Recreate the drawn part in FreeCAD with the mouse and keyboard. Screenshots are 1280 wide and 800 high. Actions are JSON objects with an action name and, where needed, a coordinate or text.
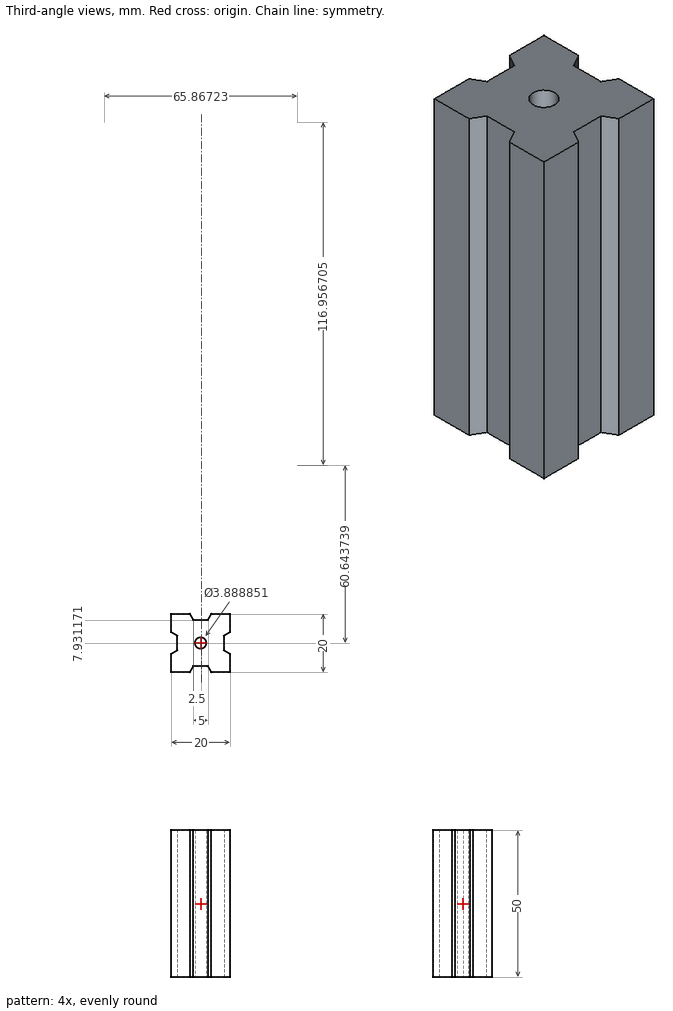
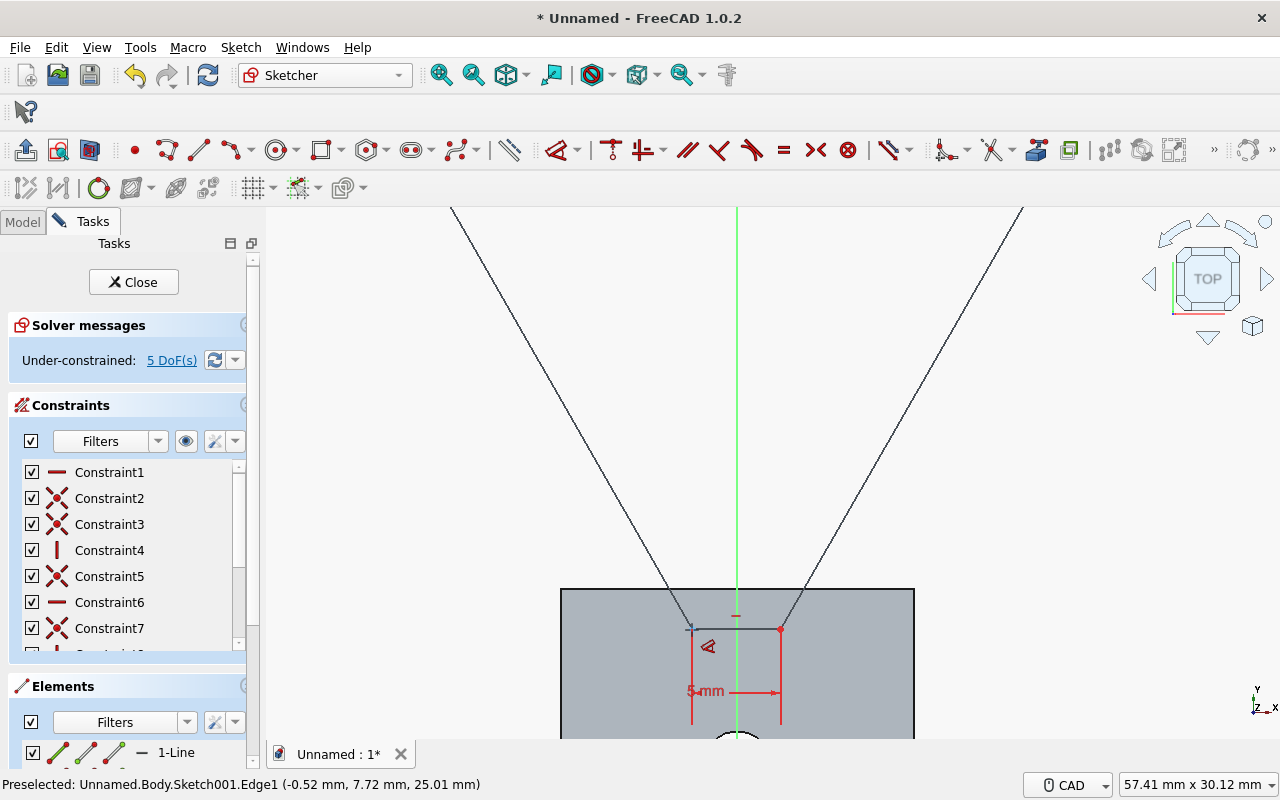
{"action": "left_click", "coordinate": [692, 629]}
{"action": "left_click", "coordinate": [715, 595]}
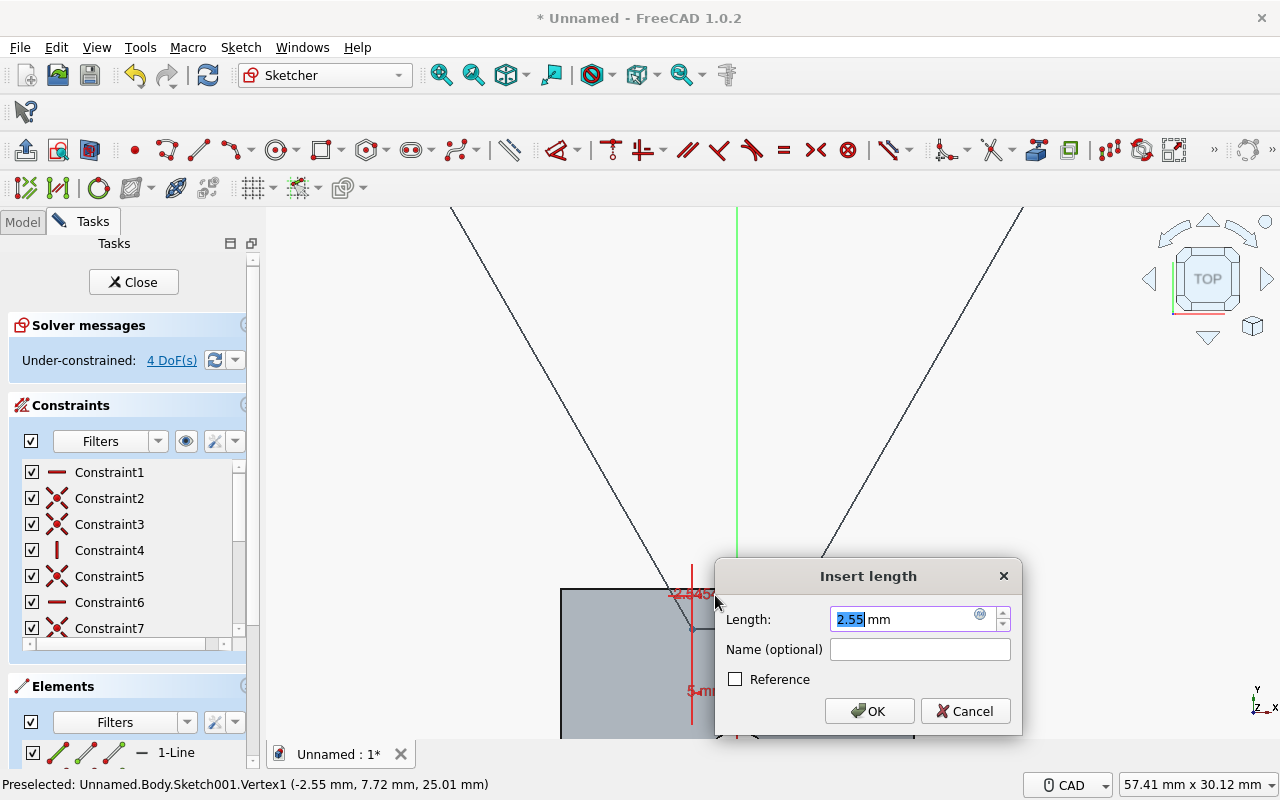
{"action": "type", "text": "2.5"}
{"action": "key", "text": "Return"}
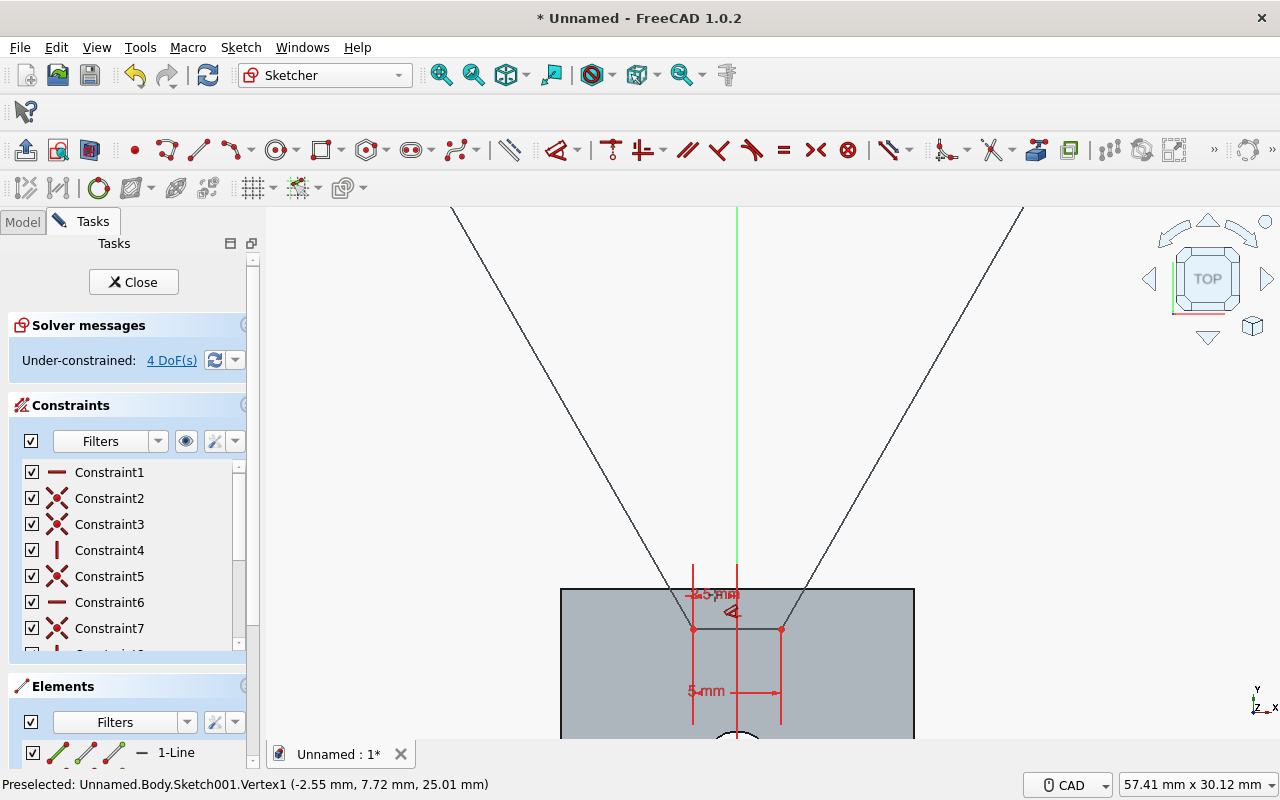
{"action": "scroll", "coordinate": [700, 632], "scroll_direction": "down", "scroll_amount": 11}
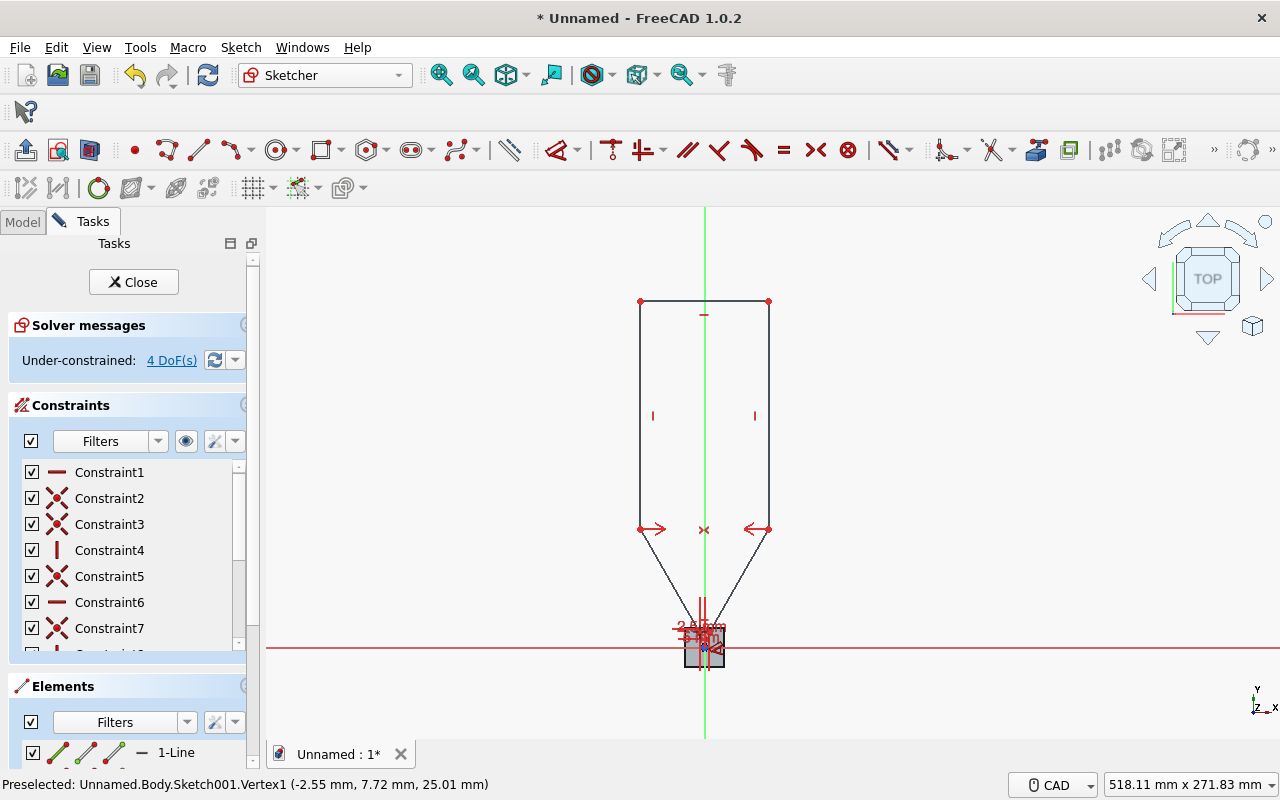
{"action": "left_click", "coordinate": [730, 301]}
{"action": "left_click", "coordinate": [675, 267]}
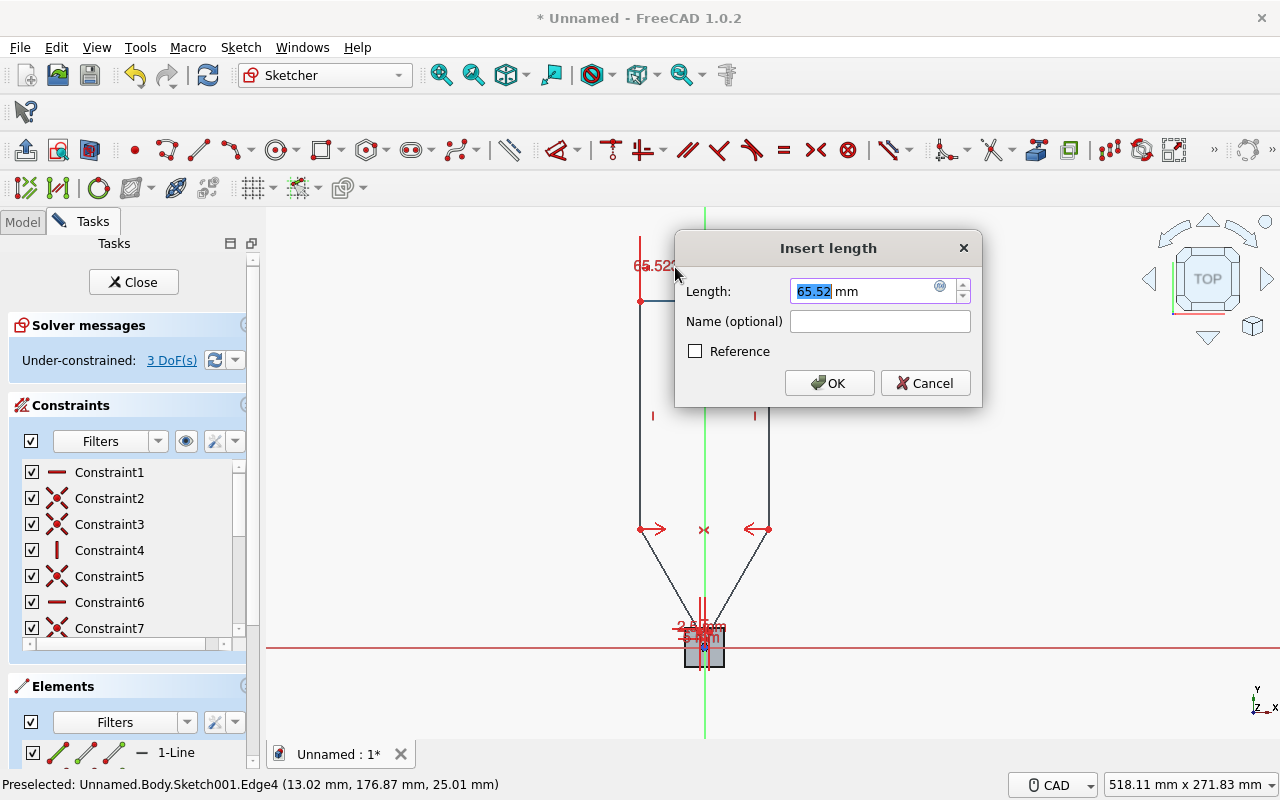
{"action": "type", "text": "65.86723"}
{"action": "key", "text": "Return"}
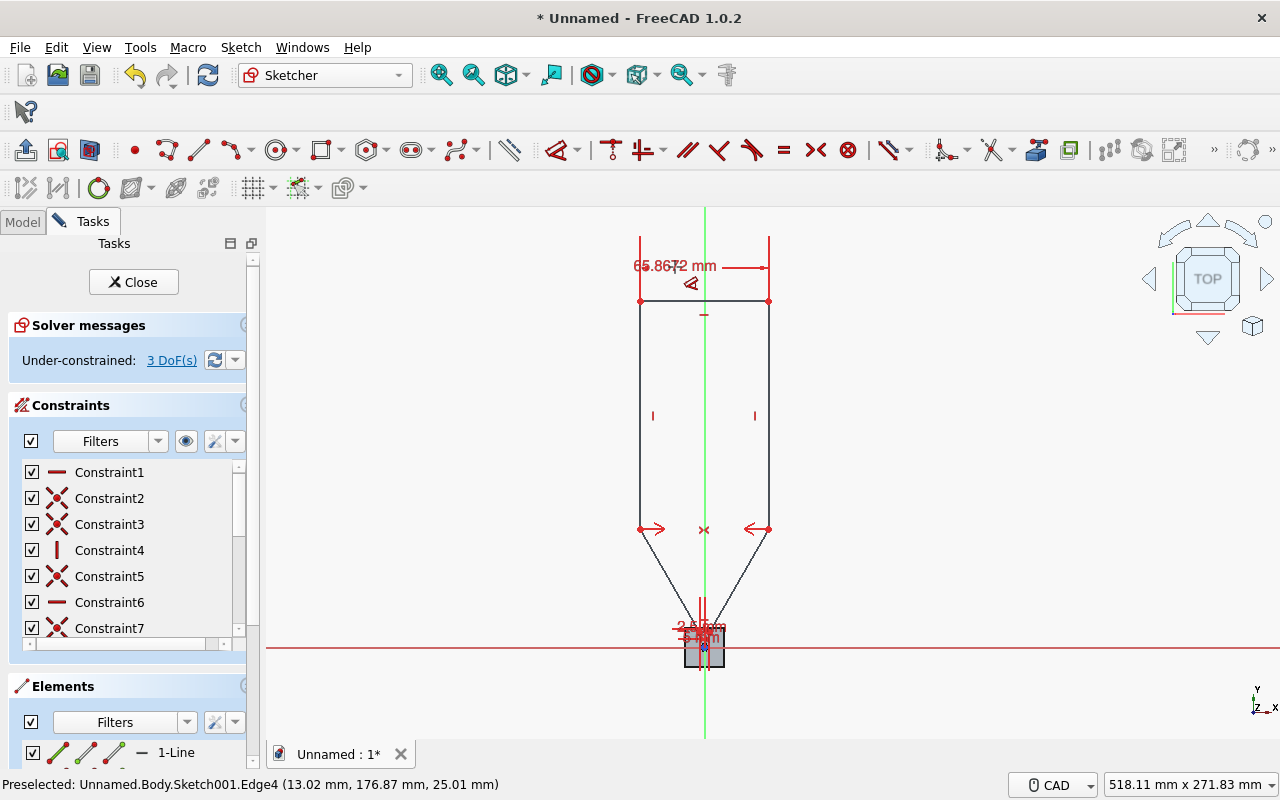
{"action": "scroll", "coordinate": [700, 632], "scroll_direction": "up", "scroll_amount": 5}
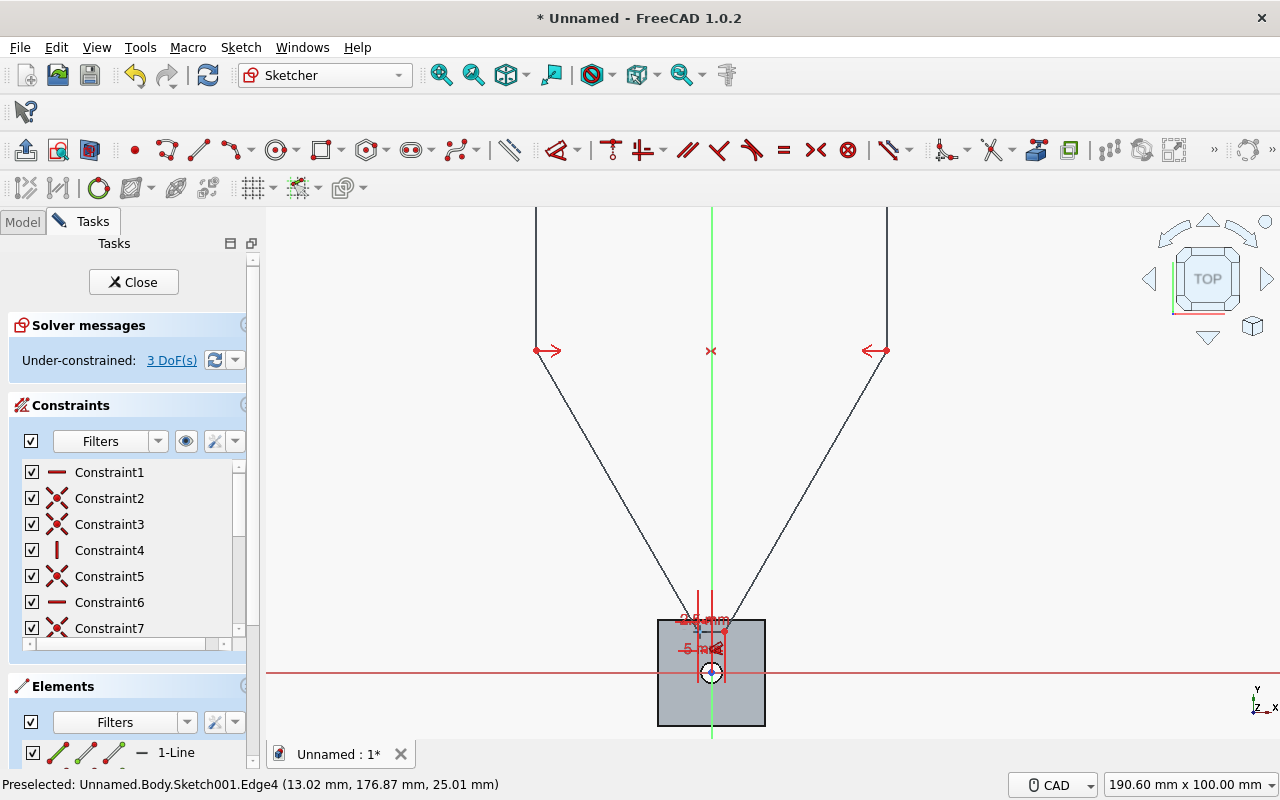
{"action": "left_click", "coordinate": [698, 632]}
{"action": "left_click", "coordinate": [616, 652]}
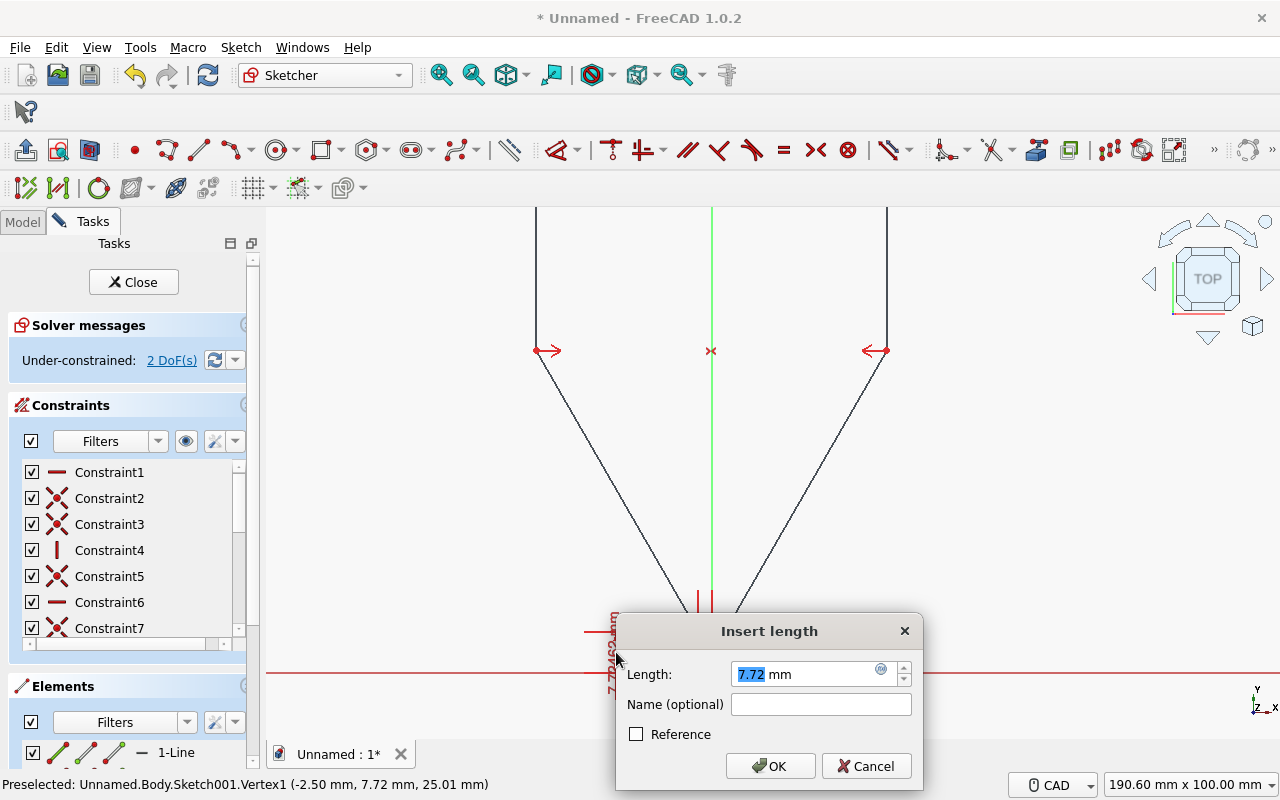
{"action": "type", "text": "7.931171"}
{"action": "key", "text": "Return"}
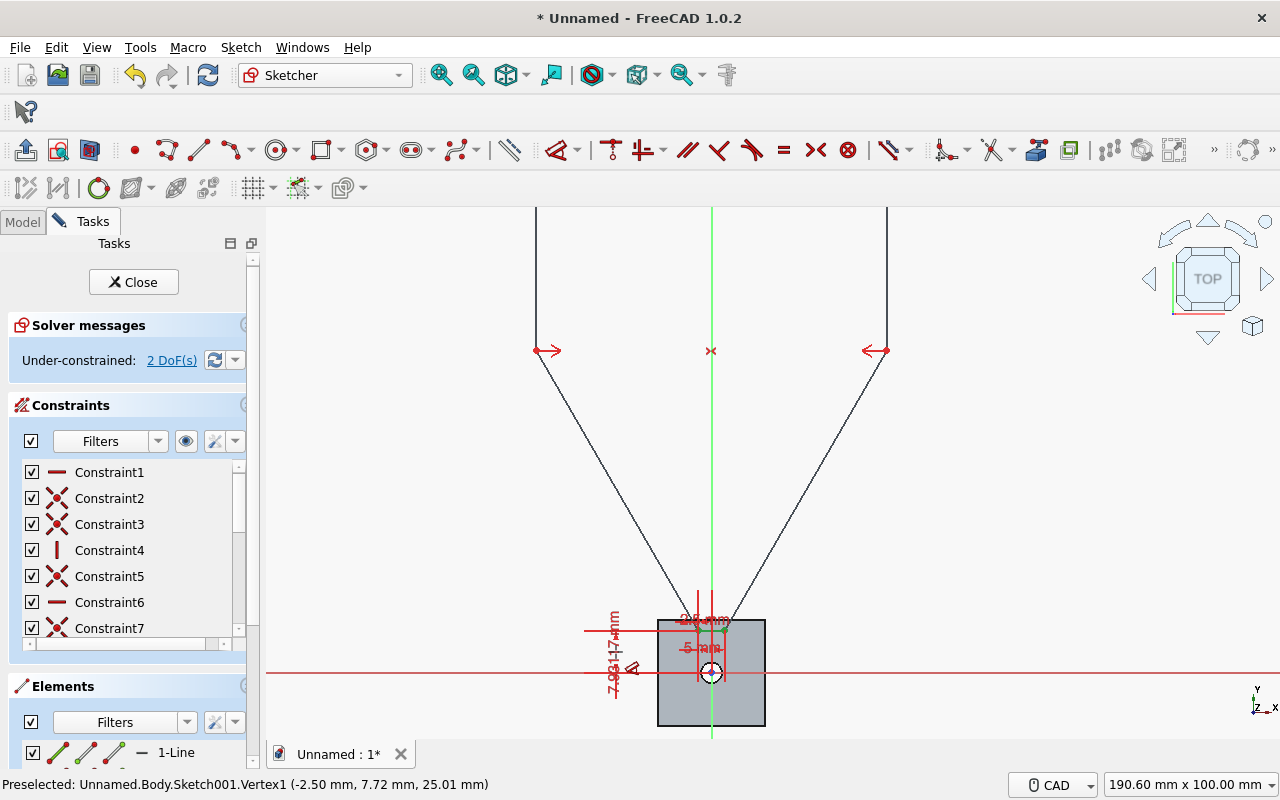
{"action": "scroll", "coordinate": [700, 632], "scroll_direction": "down", "scroll_amount": 5}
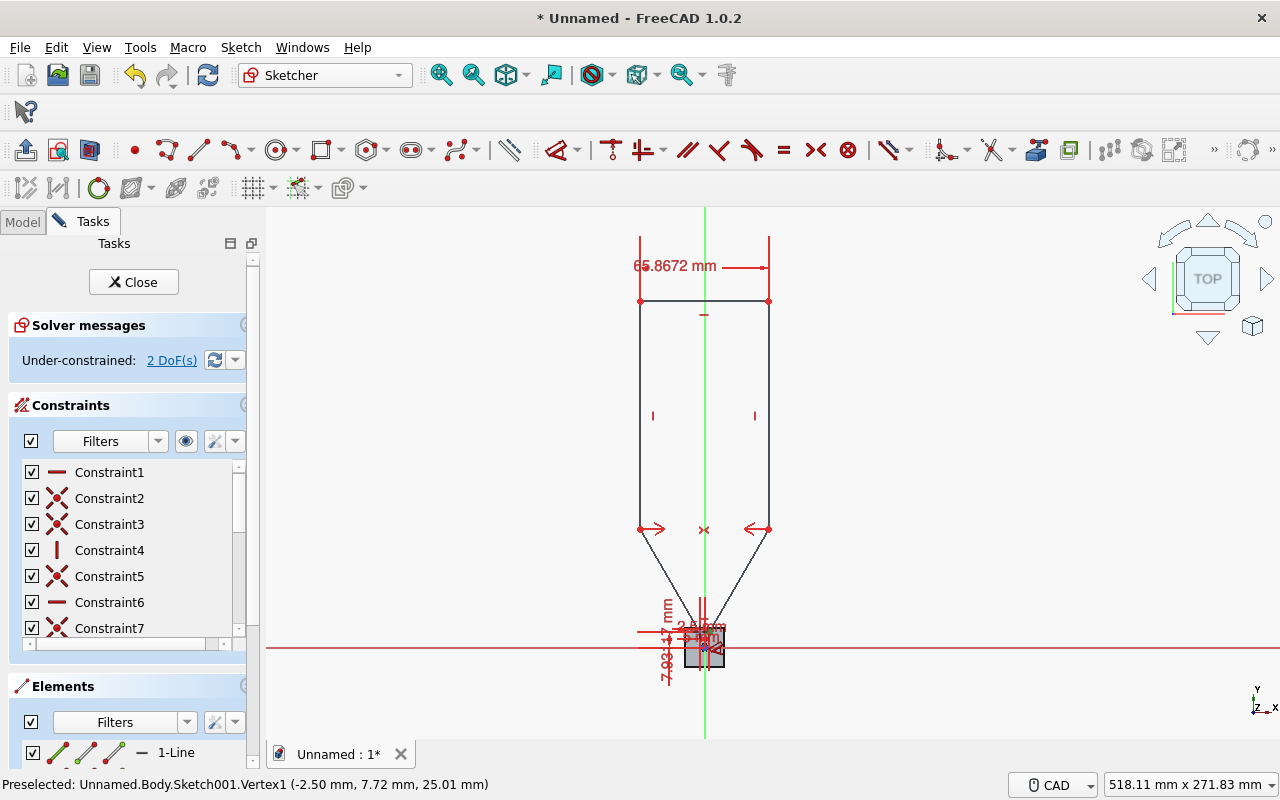
{"action": "left_click", "coordinate": [769, 461]}
{"action": "left_click", "coordinate": [803, 415]}